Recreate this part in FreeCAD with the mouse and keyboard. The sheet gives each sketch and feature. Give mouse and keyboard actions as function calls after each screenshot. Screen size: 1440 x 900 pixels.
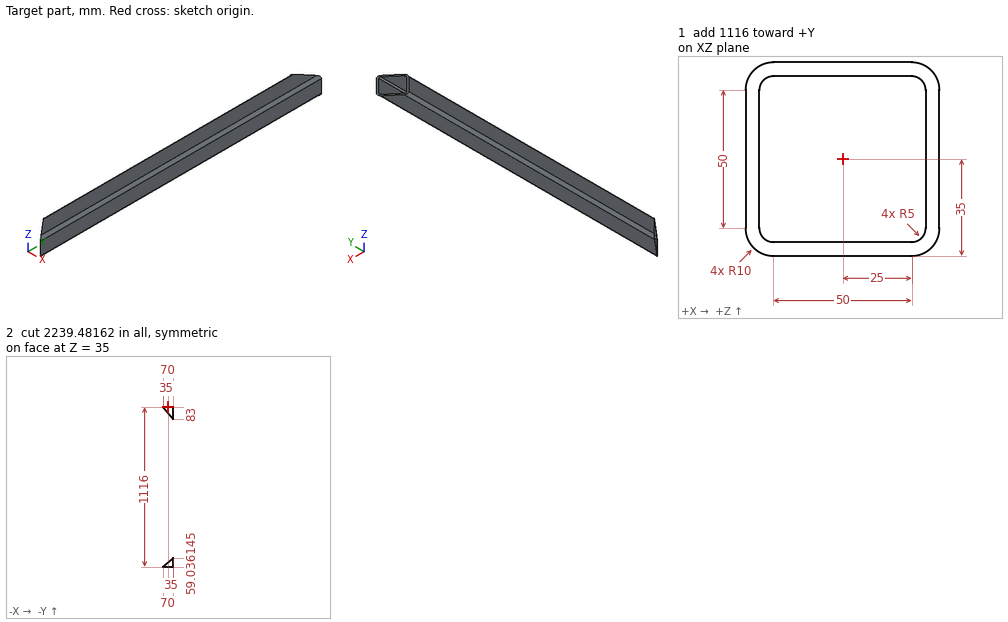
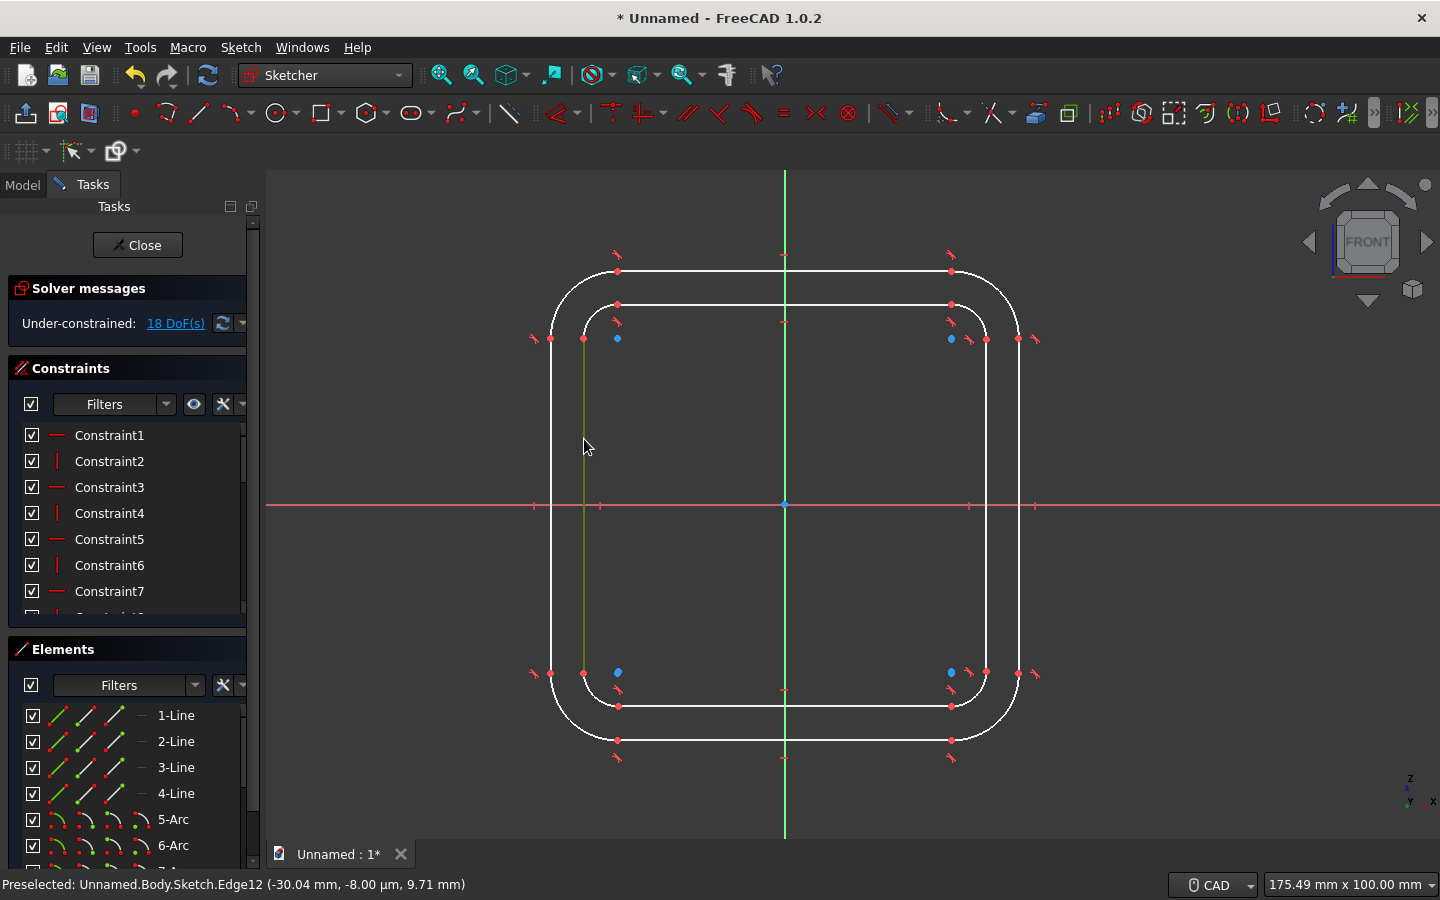
click(602, 308)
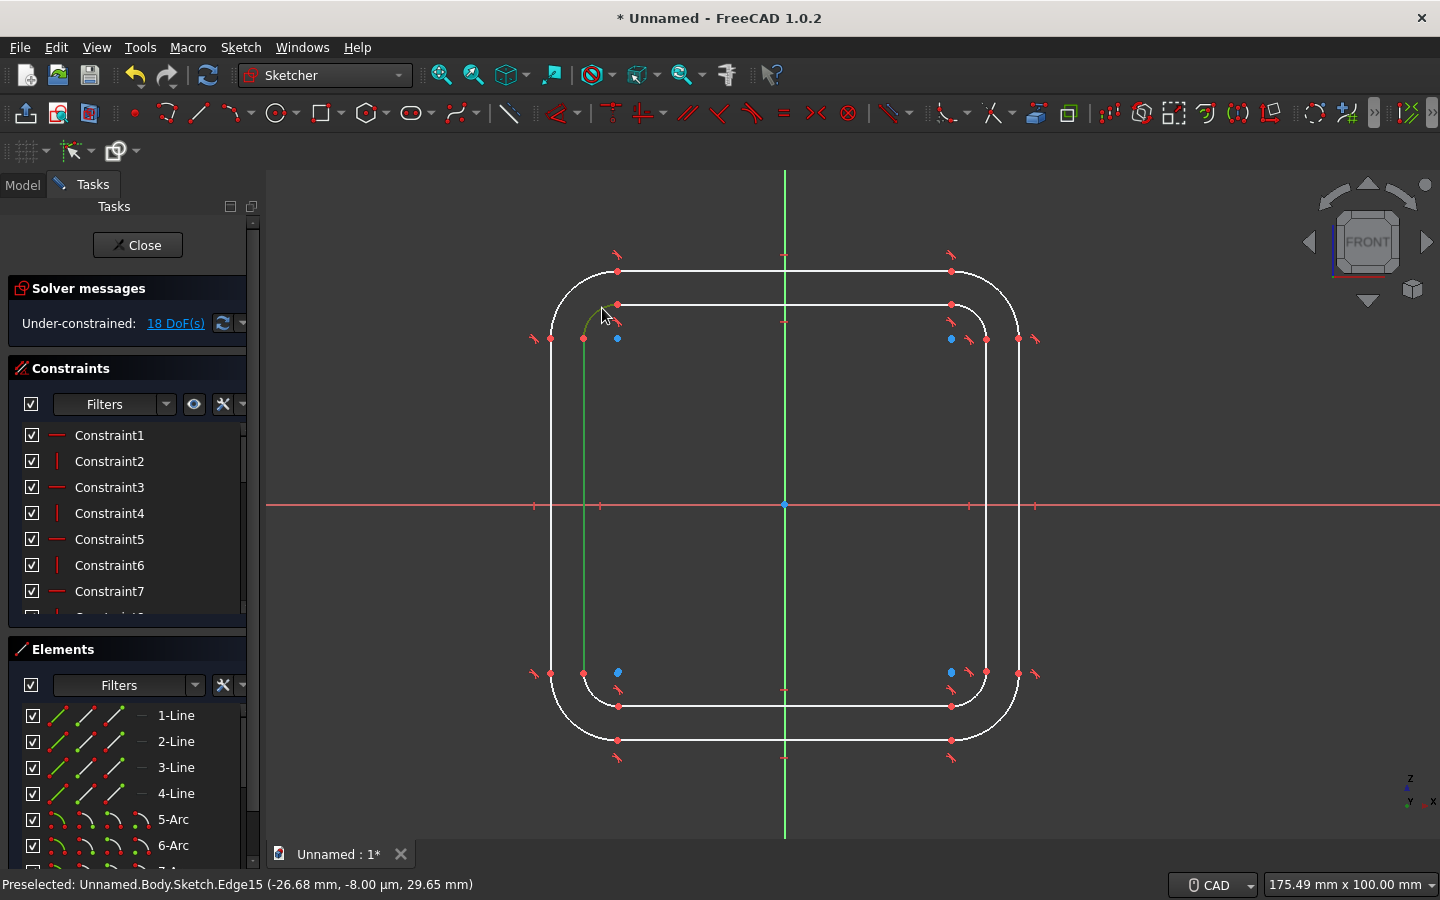
key(t)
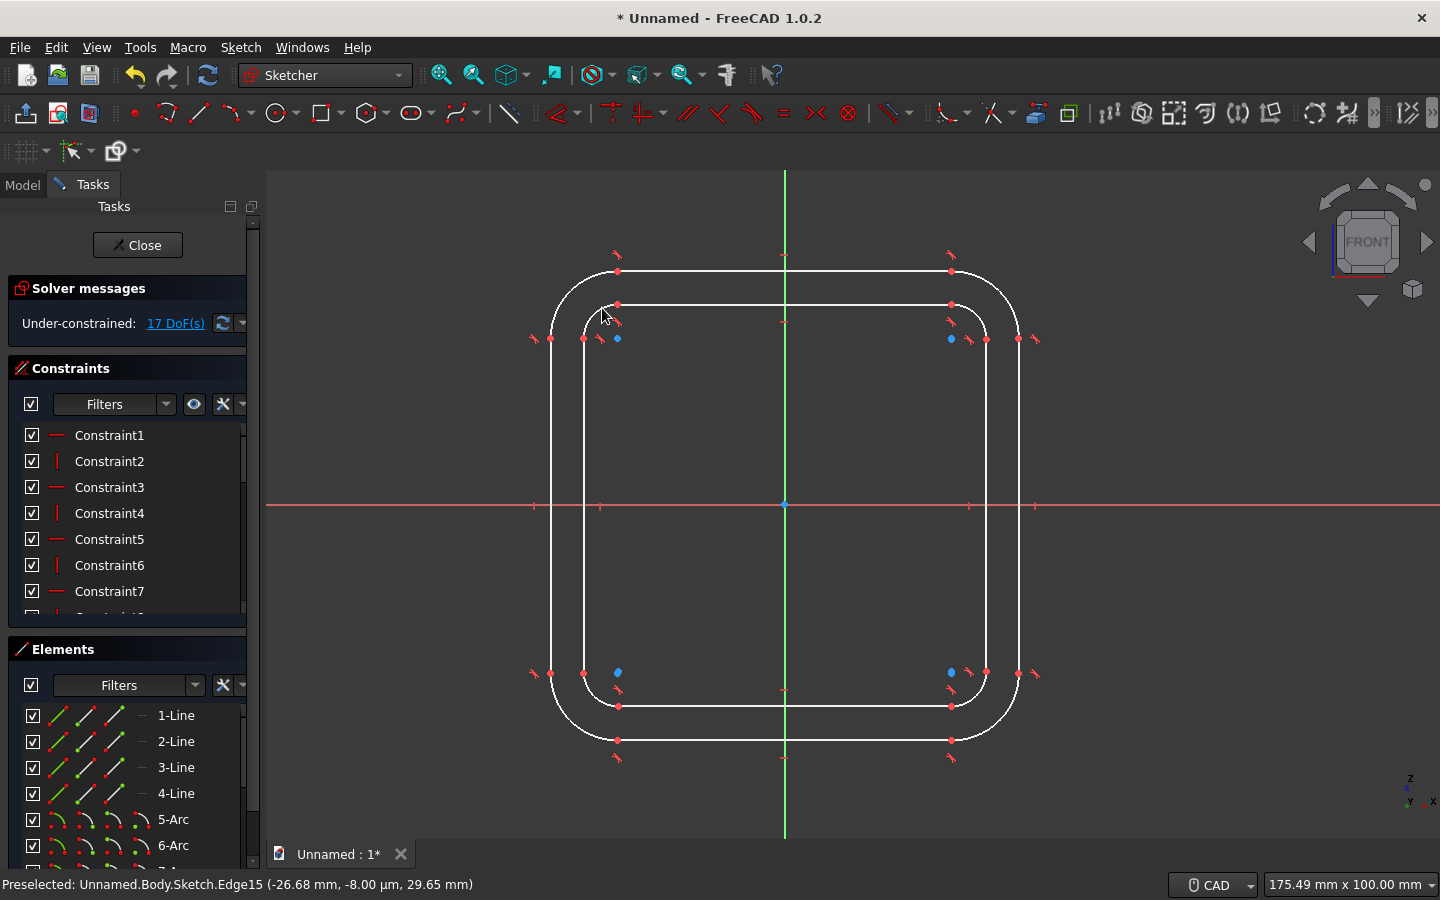
click(584, 439)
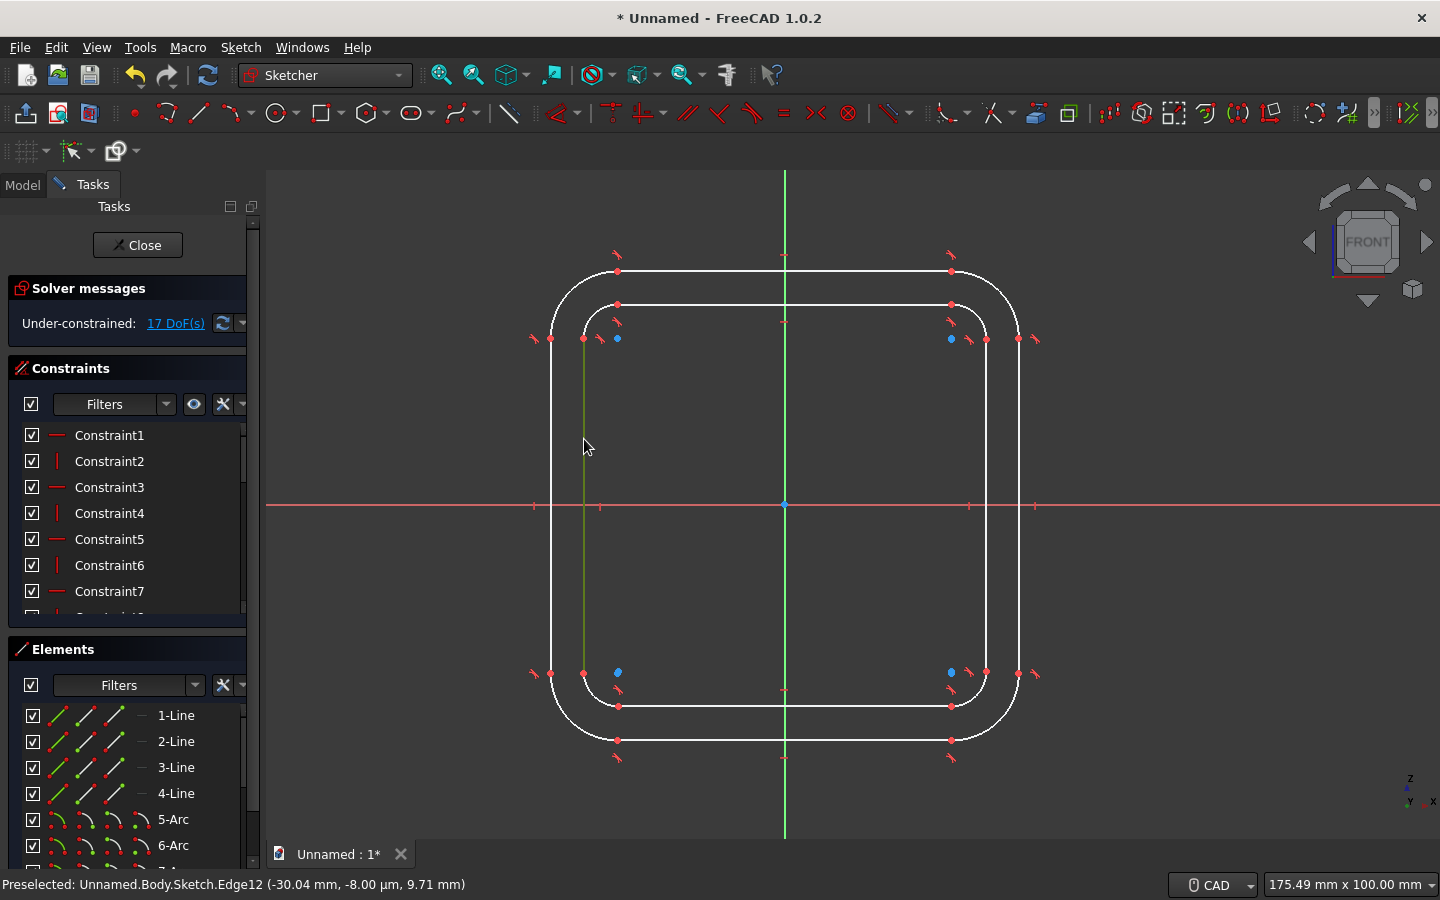
click(588, 689)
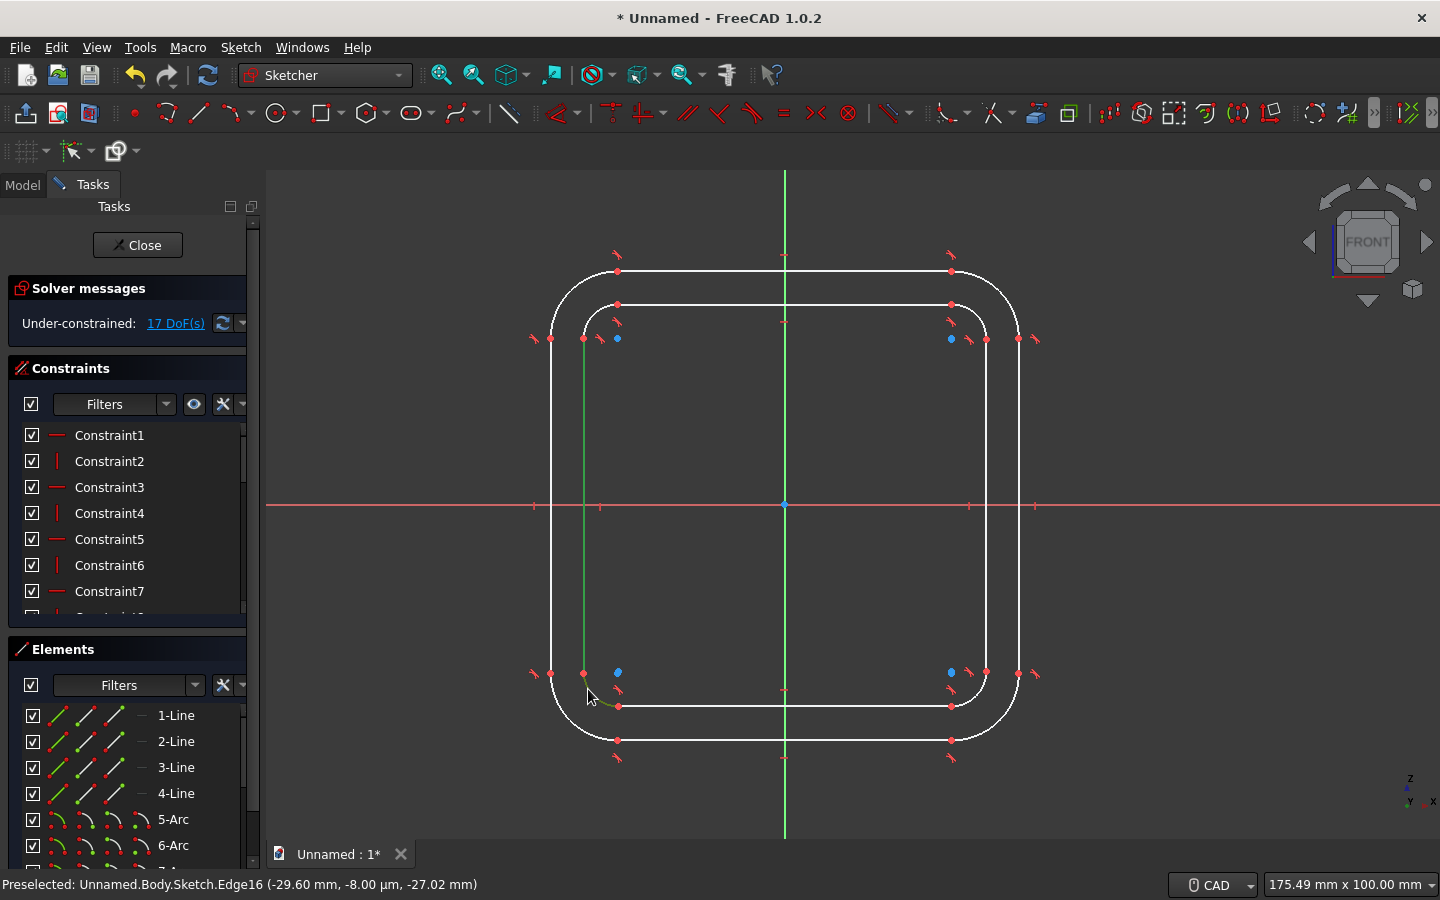
key(t)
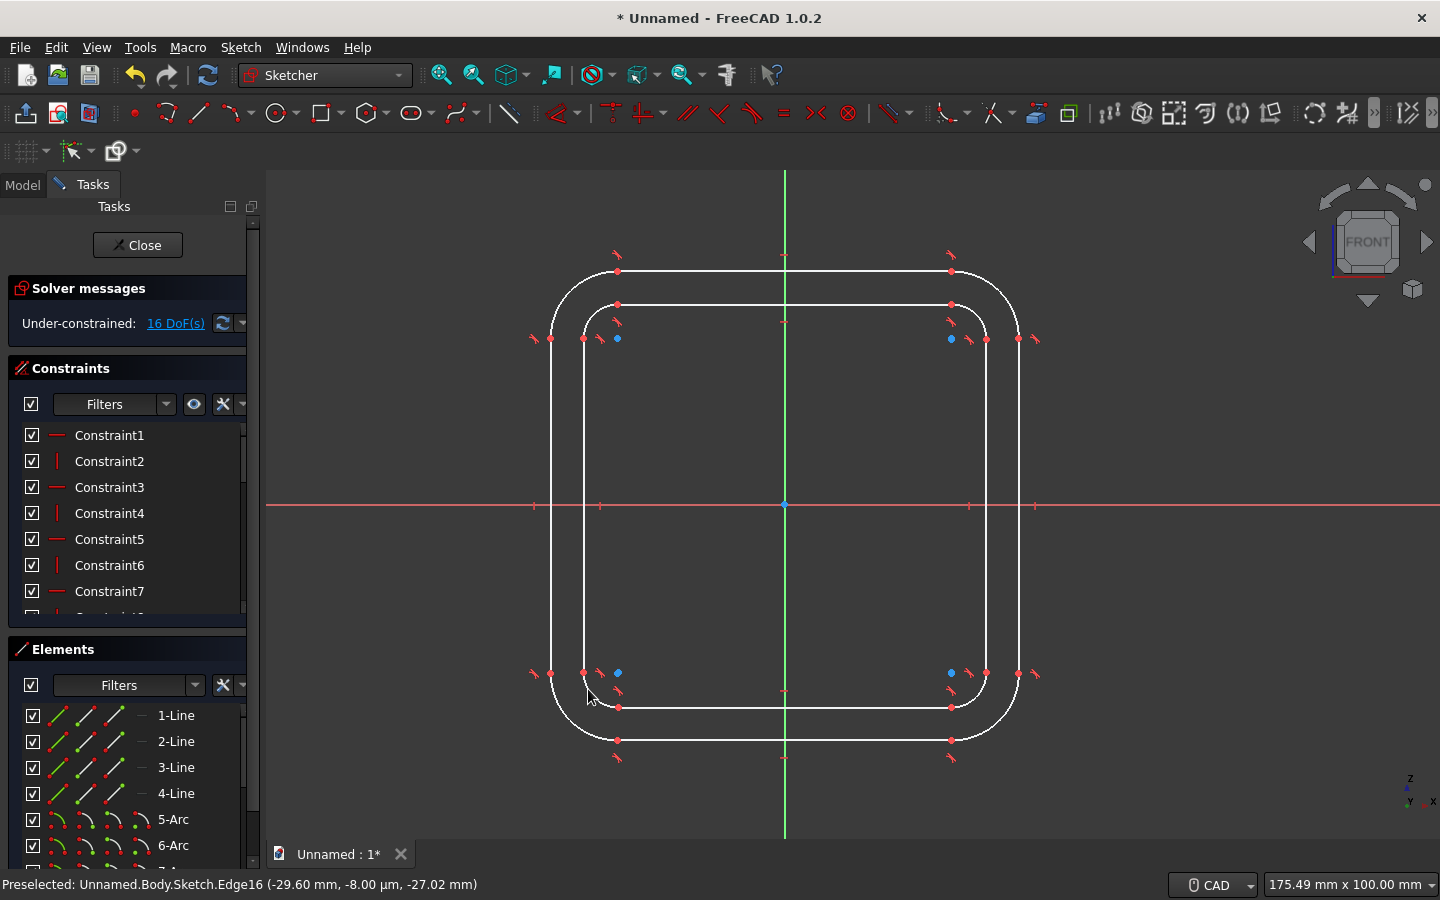
click(982, 733)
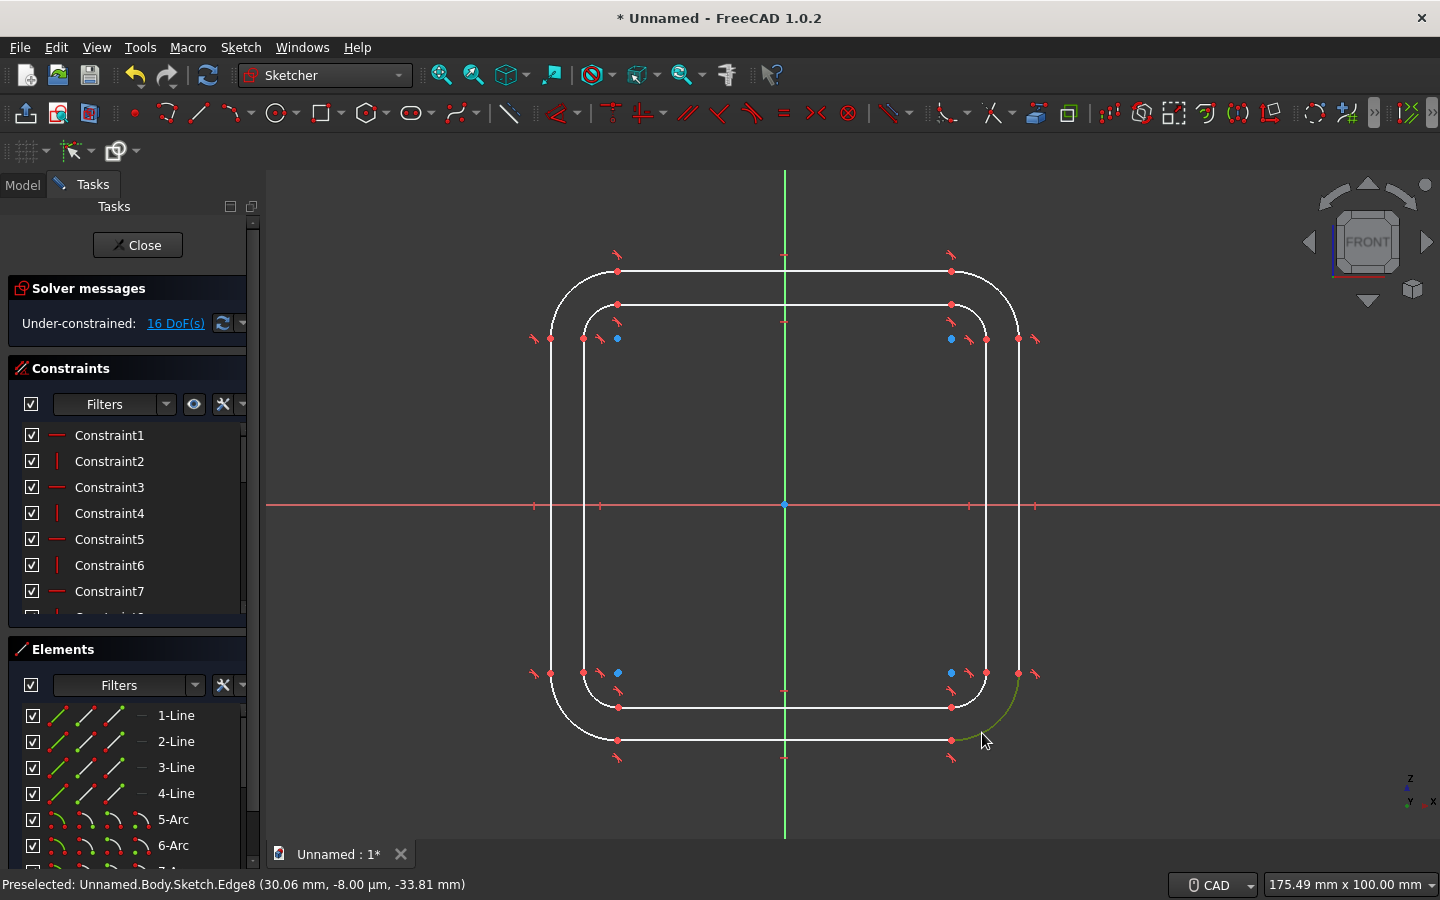
click(967, 704)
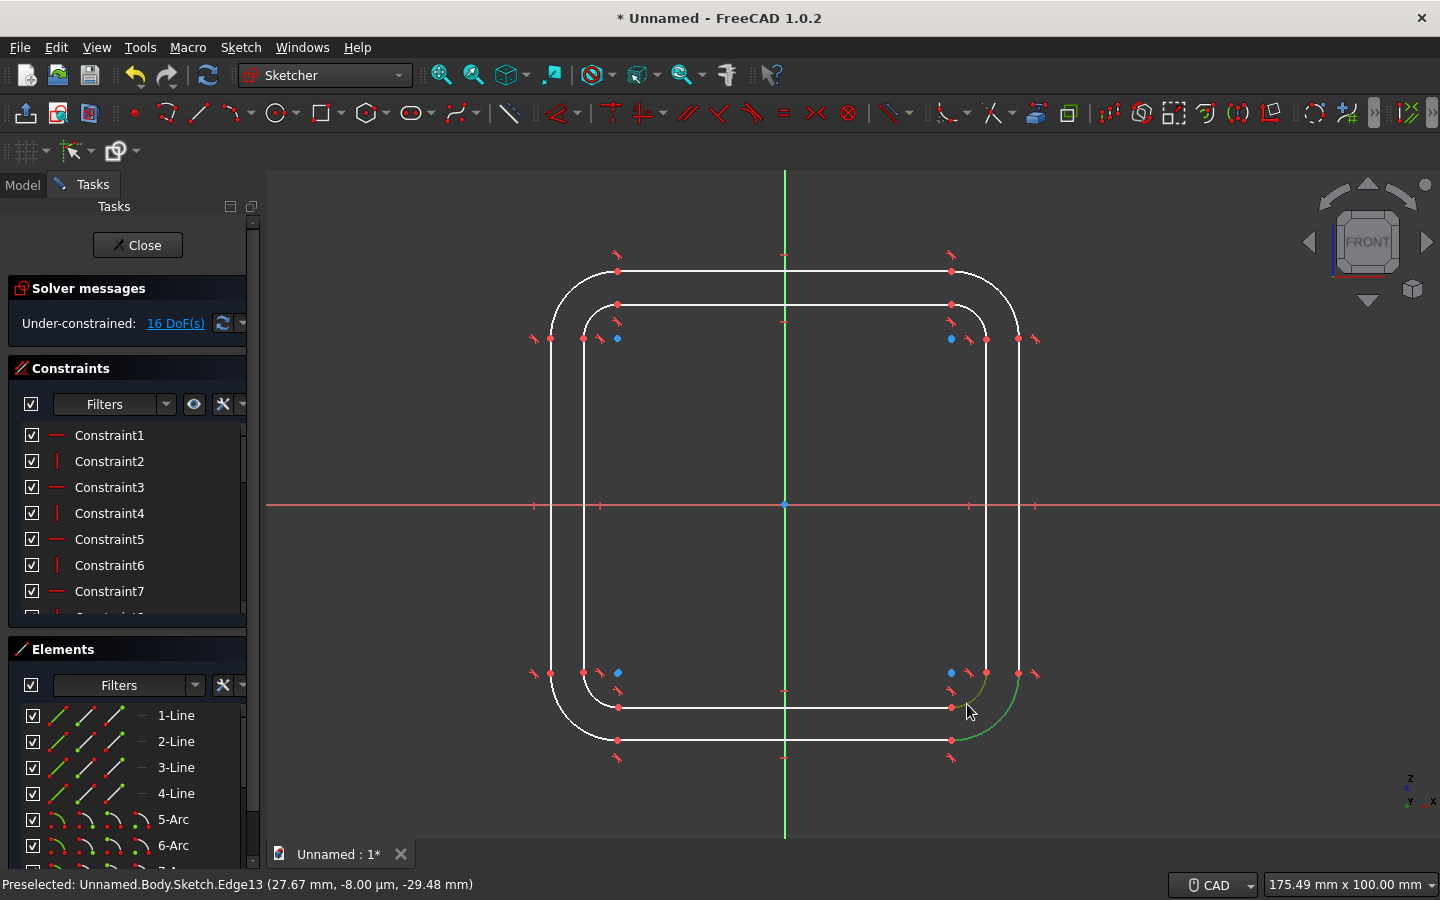
key(c)